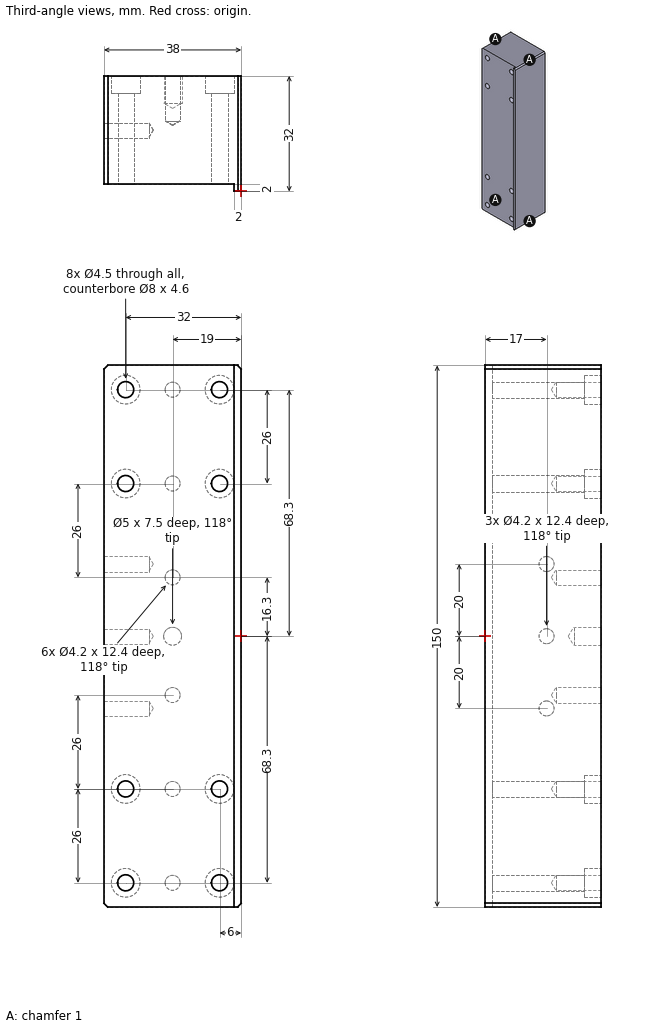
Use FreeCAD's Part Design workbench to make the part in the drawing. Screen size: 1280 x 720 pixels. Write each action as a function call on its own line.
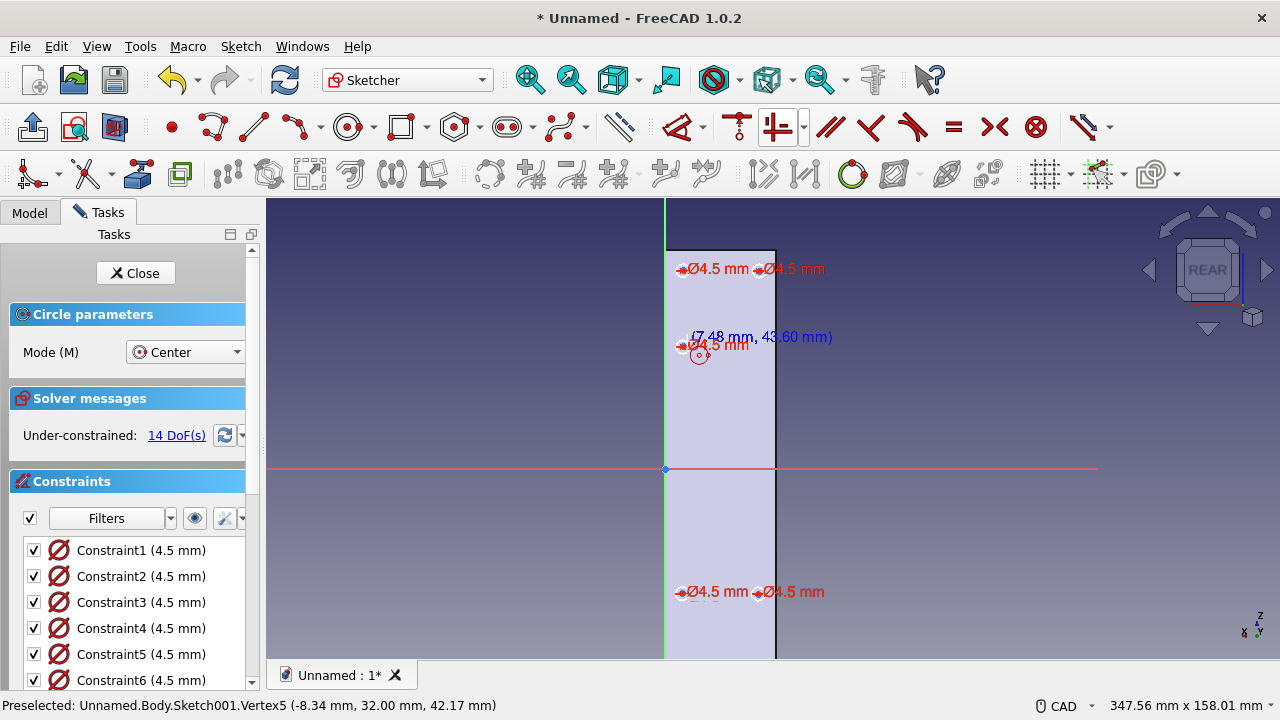
scroll(759, 346, up, 7)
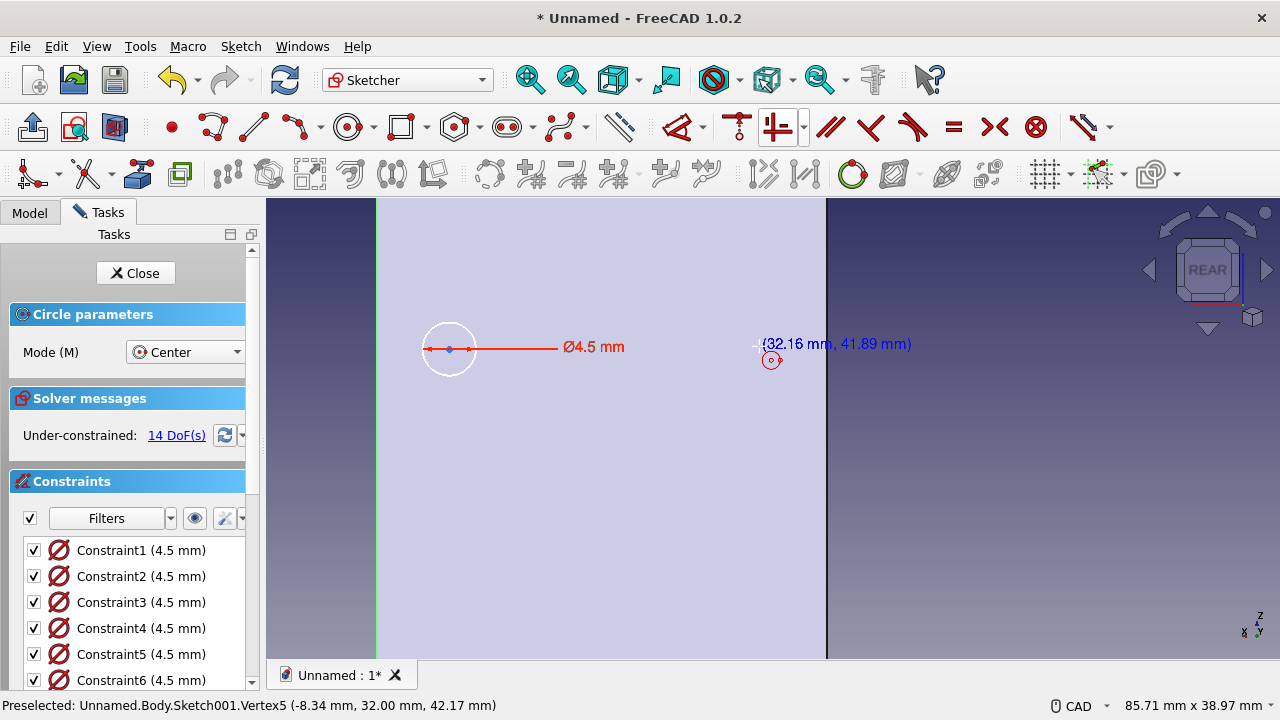
scroll(729, 346, down, 9)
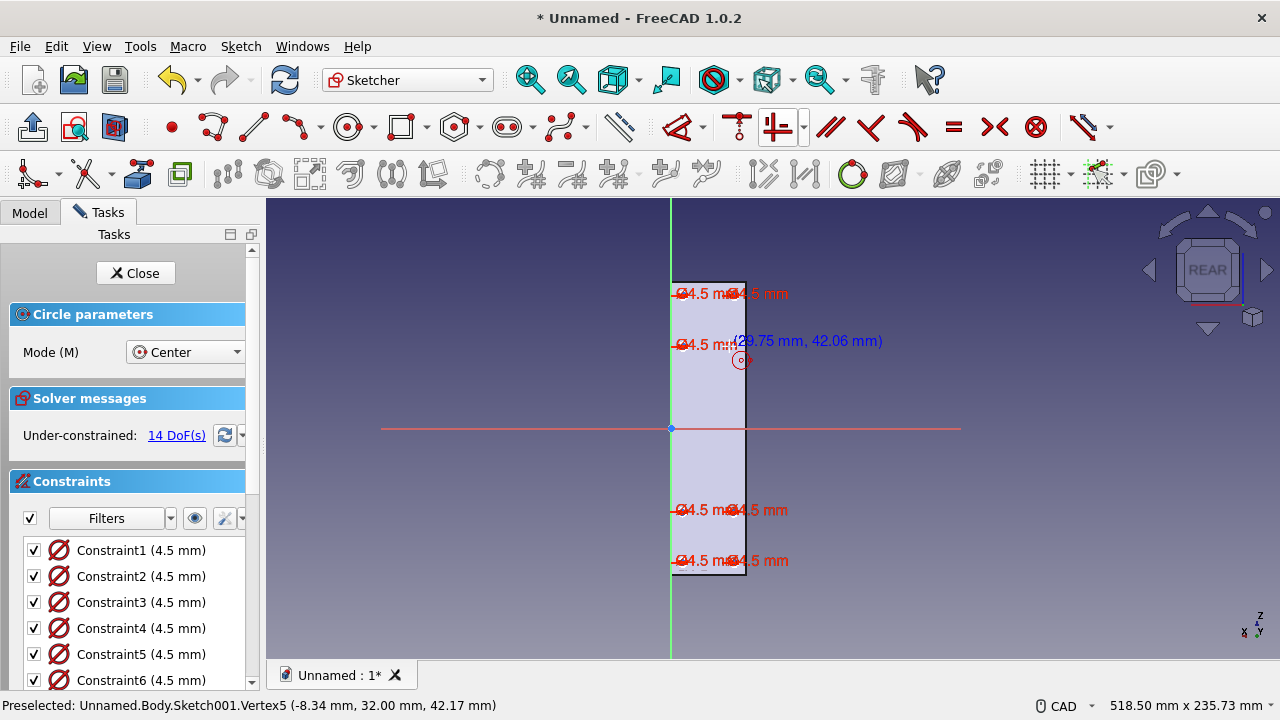
click(734, 346)
move(737, 343)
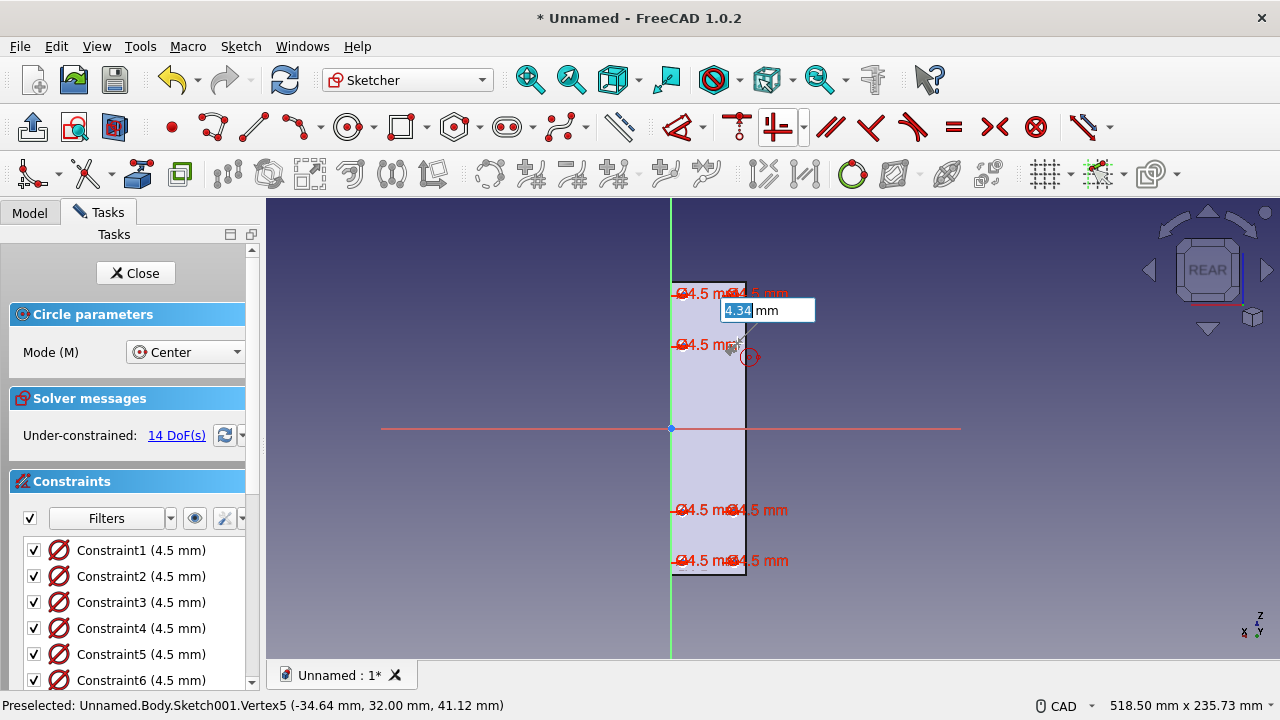
text(4.5)
key(Return)
key(Escape)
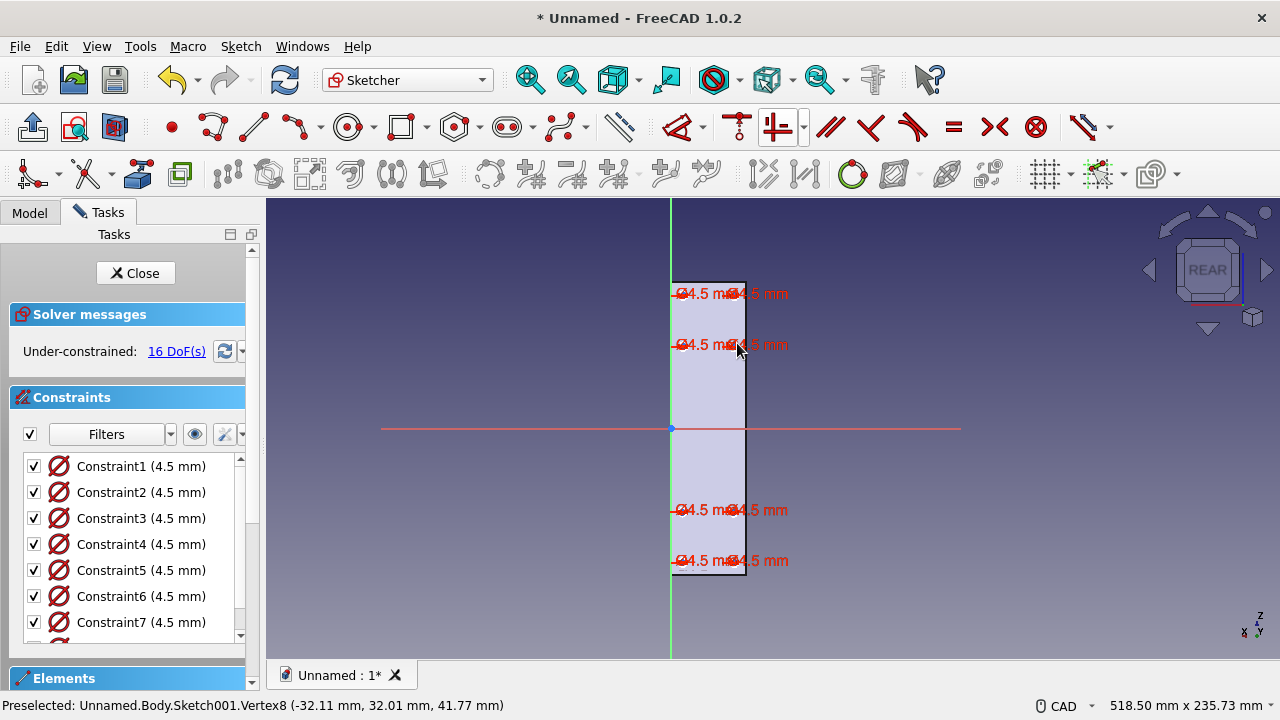
click(676, 128)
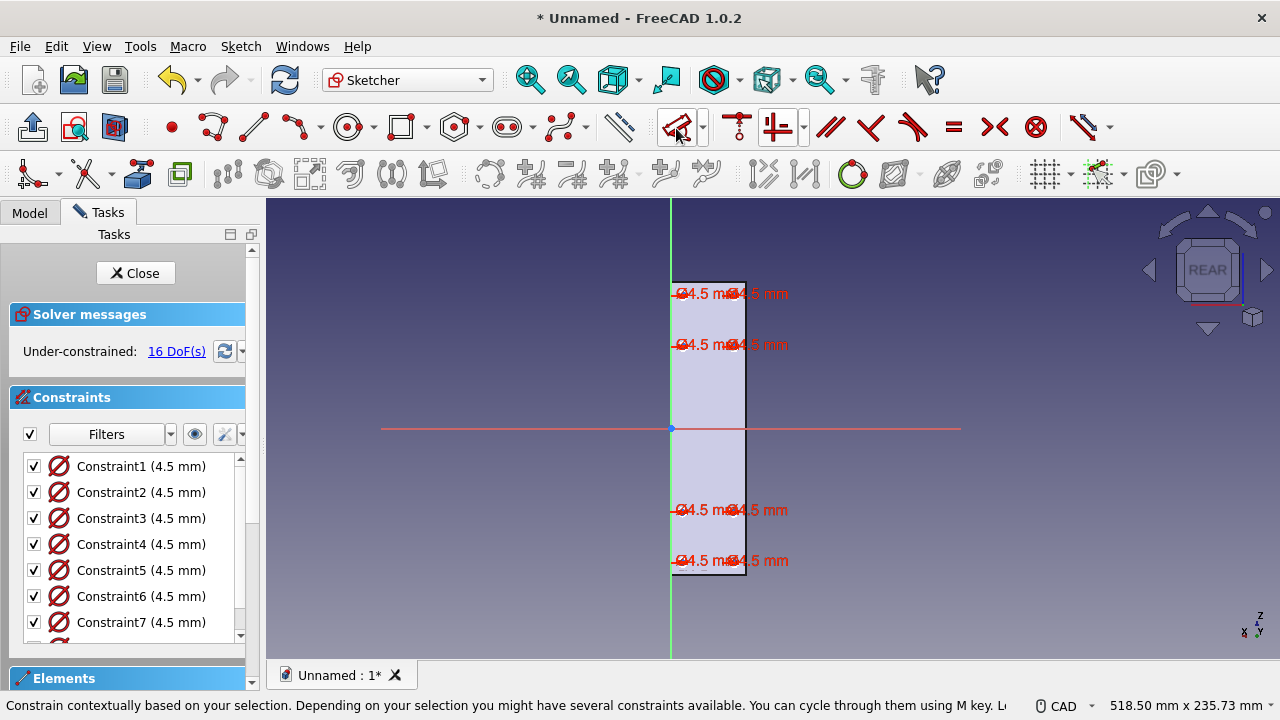
scroll(683, 512, up, 7)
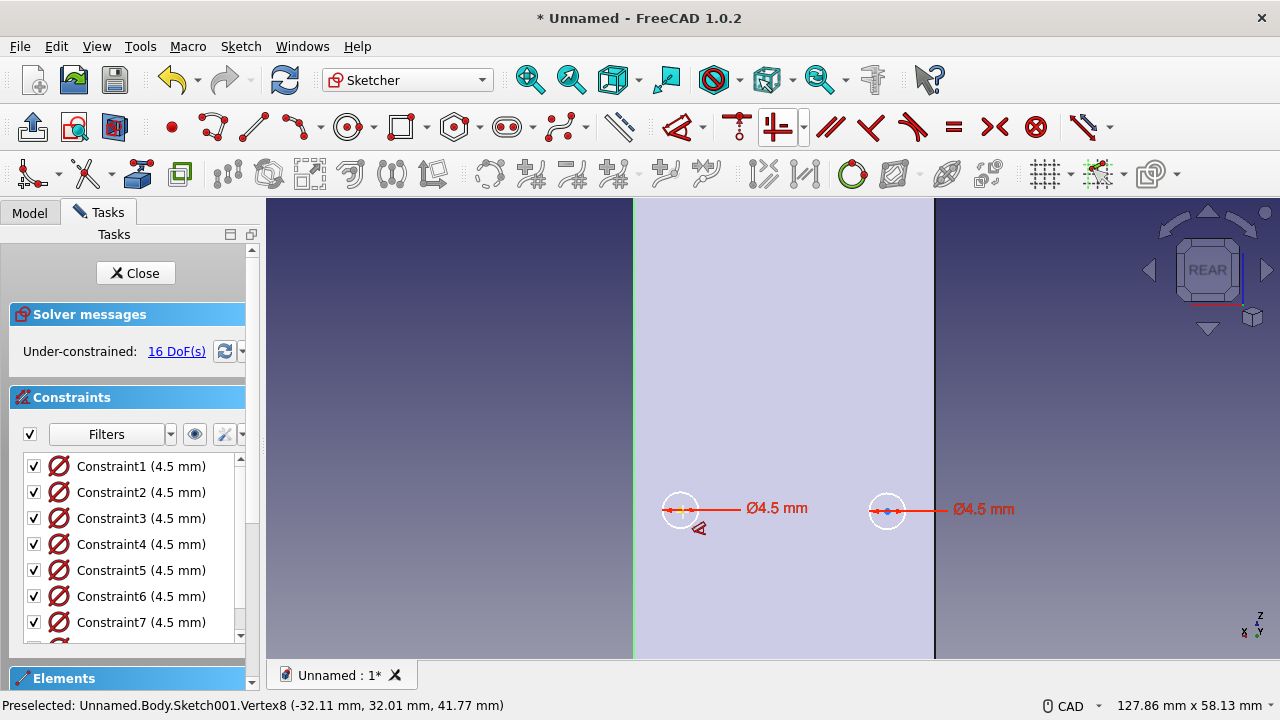
click(680, 510)
click(657, 544)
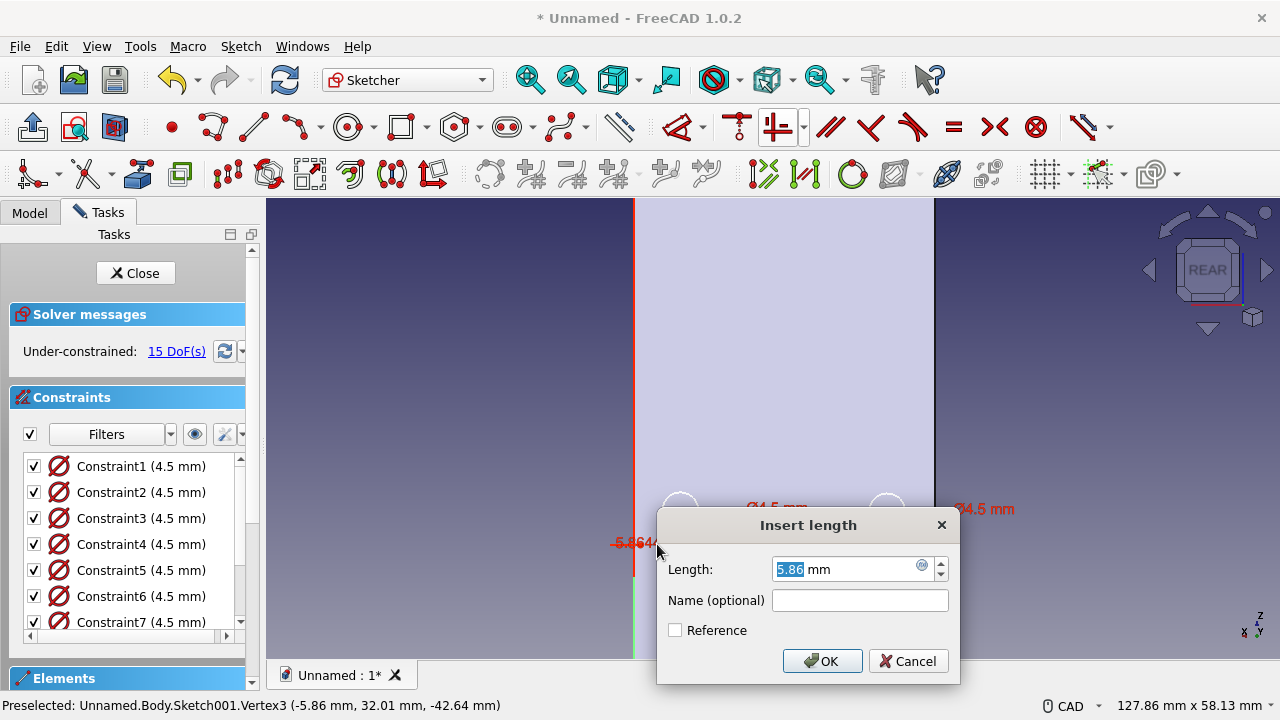
text(6)
key(Return)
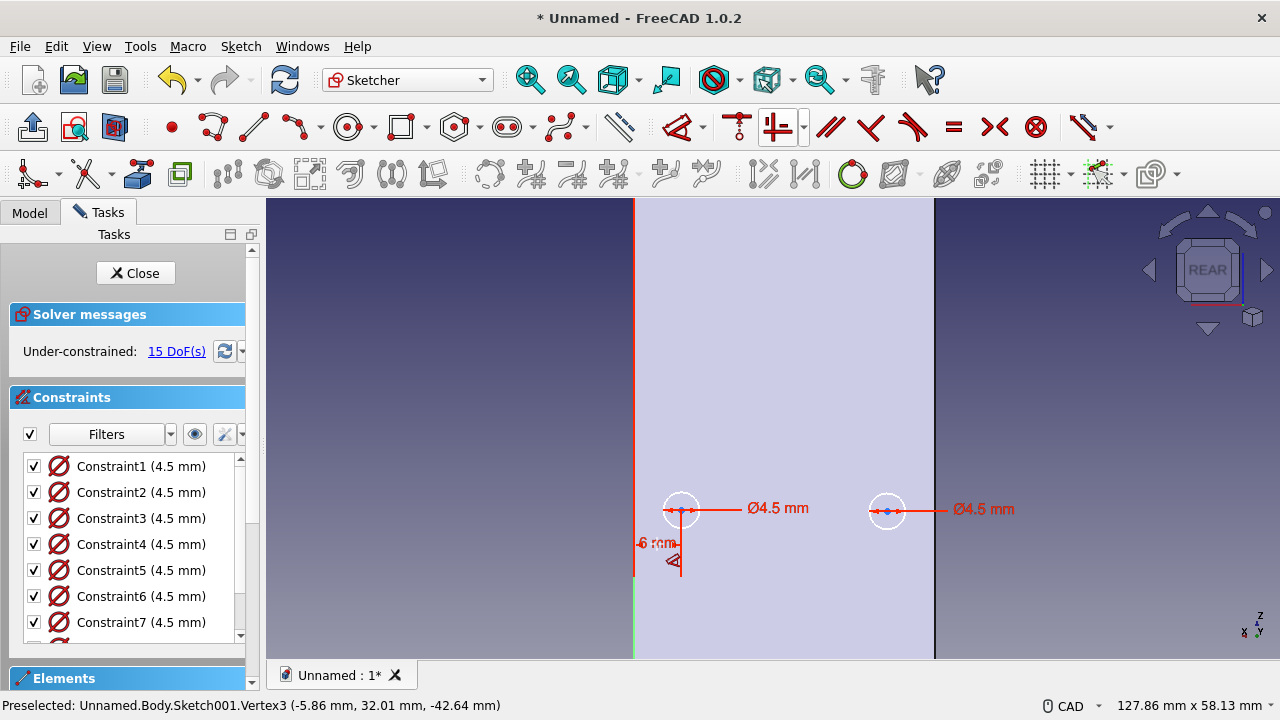
scroll(683, 512, down, 7)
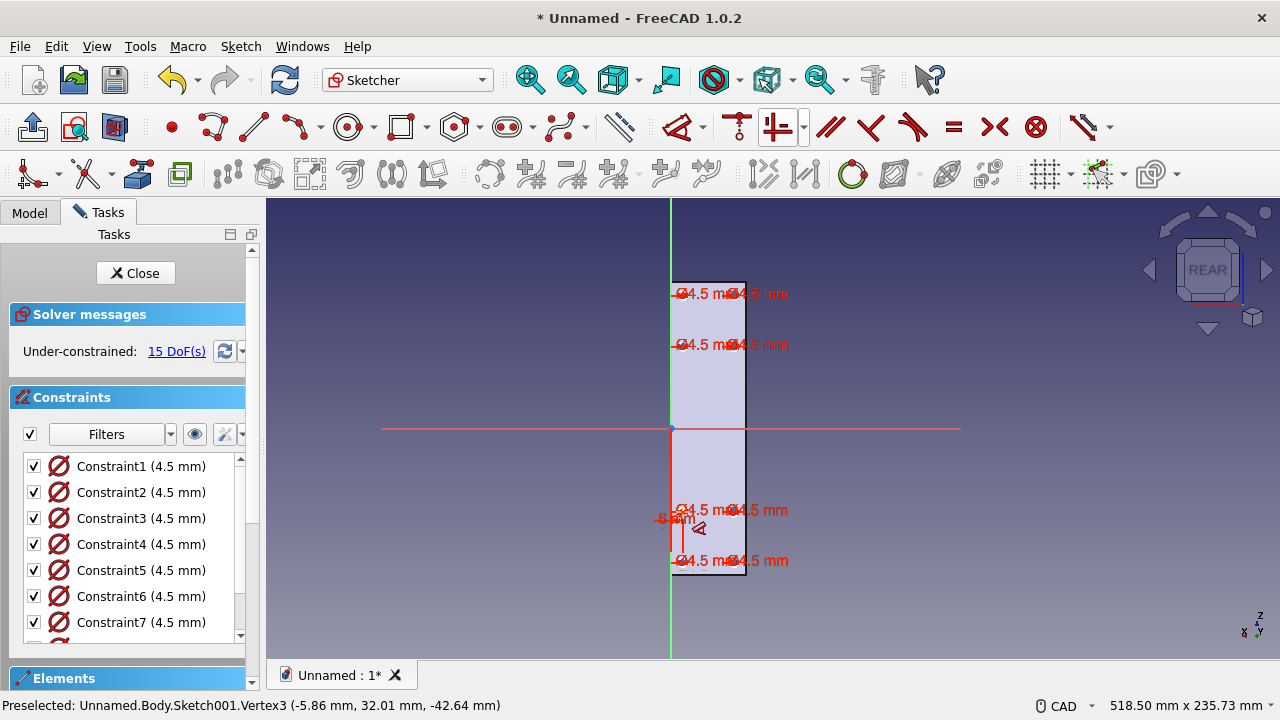
scroll(683, 563, up, 7)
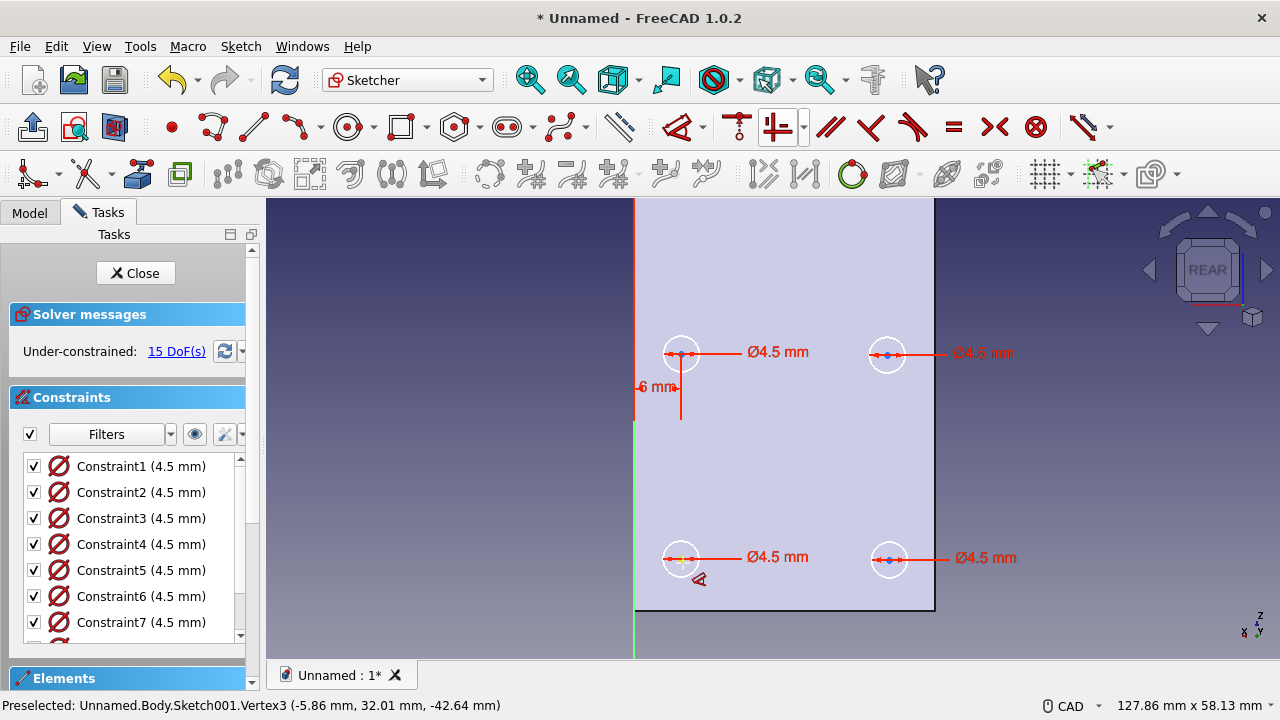
click(681, 559)
click(657, 593)